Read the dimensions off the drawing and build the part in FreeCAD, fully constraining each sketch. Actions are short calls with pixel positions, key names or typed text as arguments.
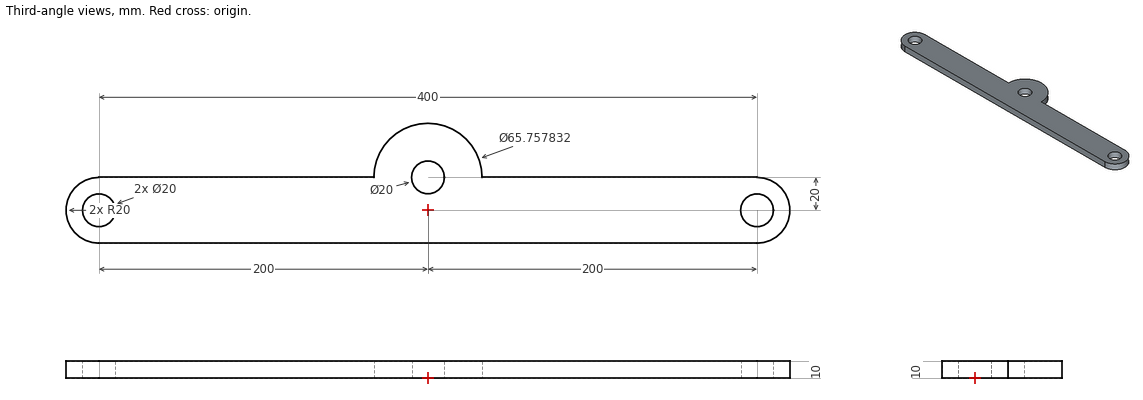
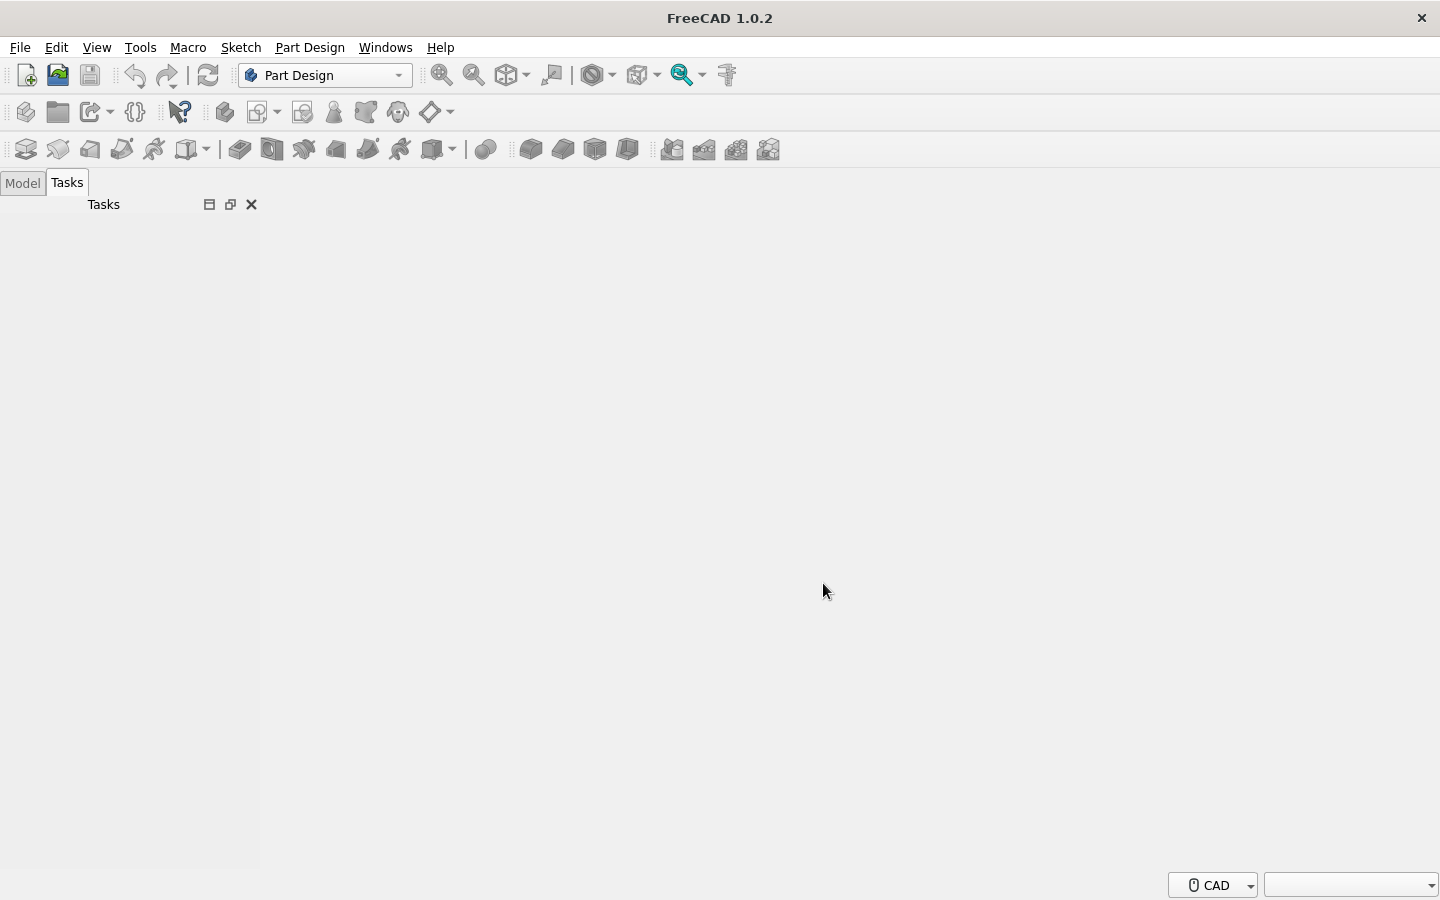
click(26, 76)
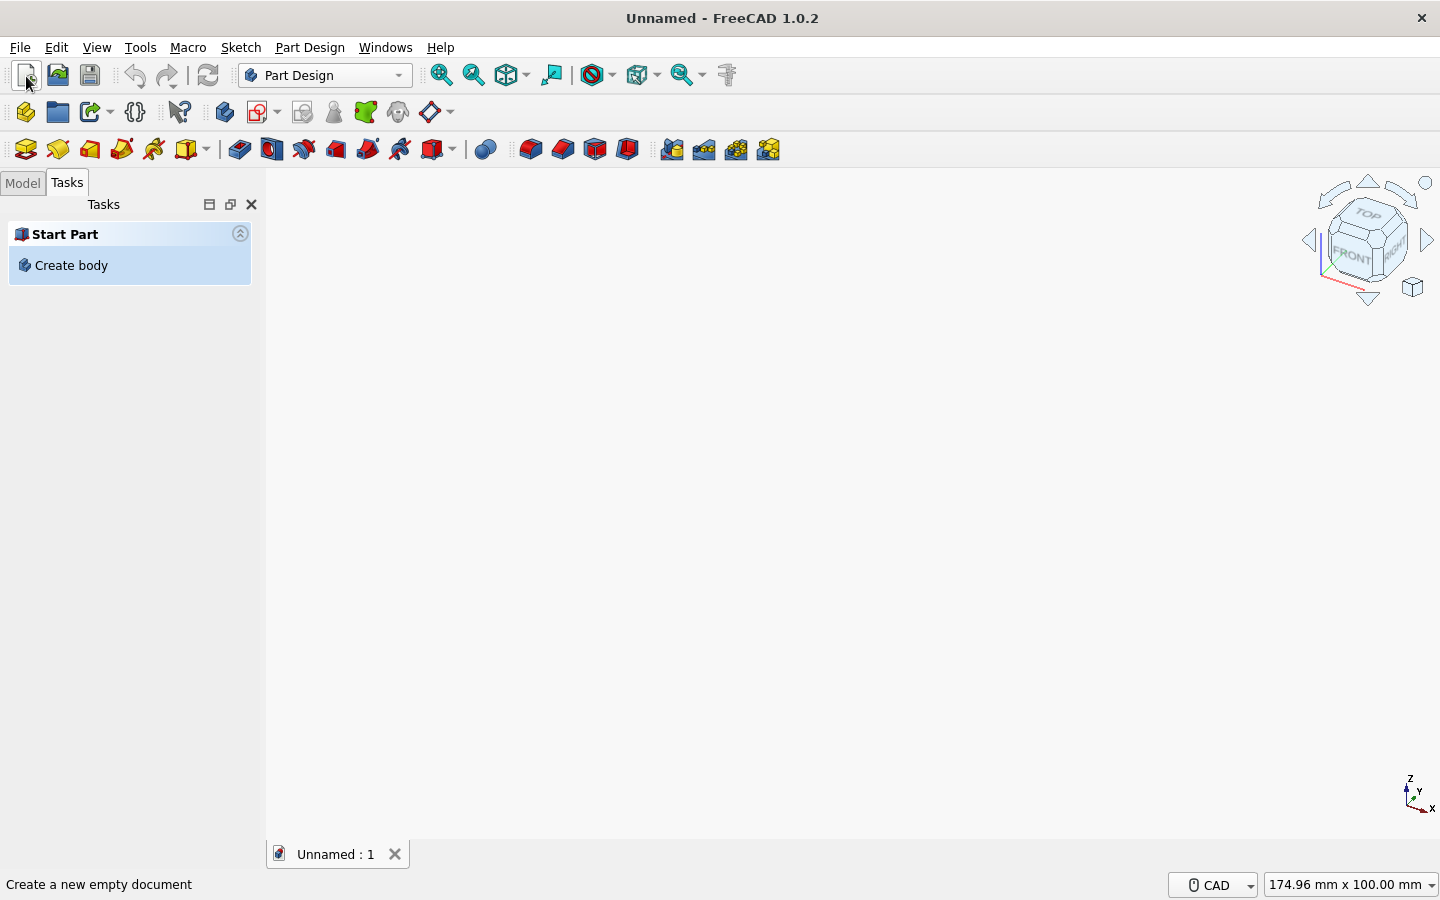
click(258, 112)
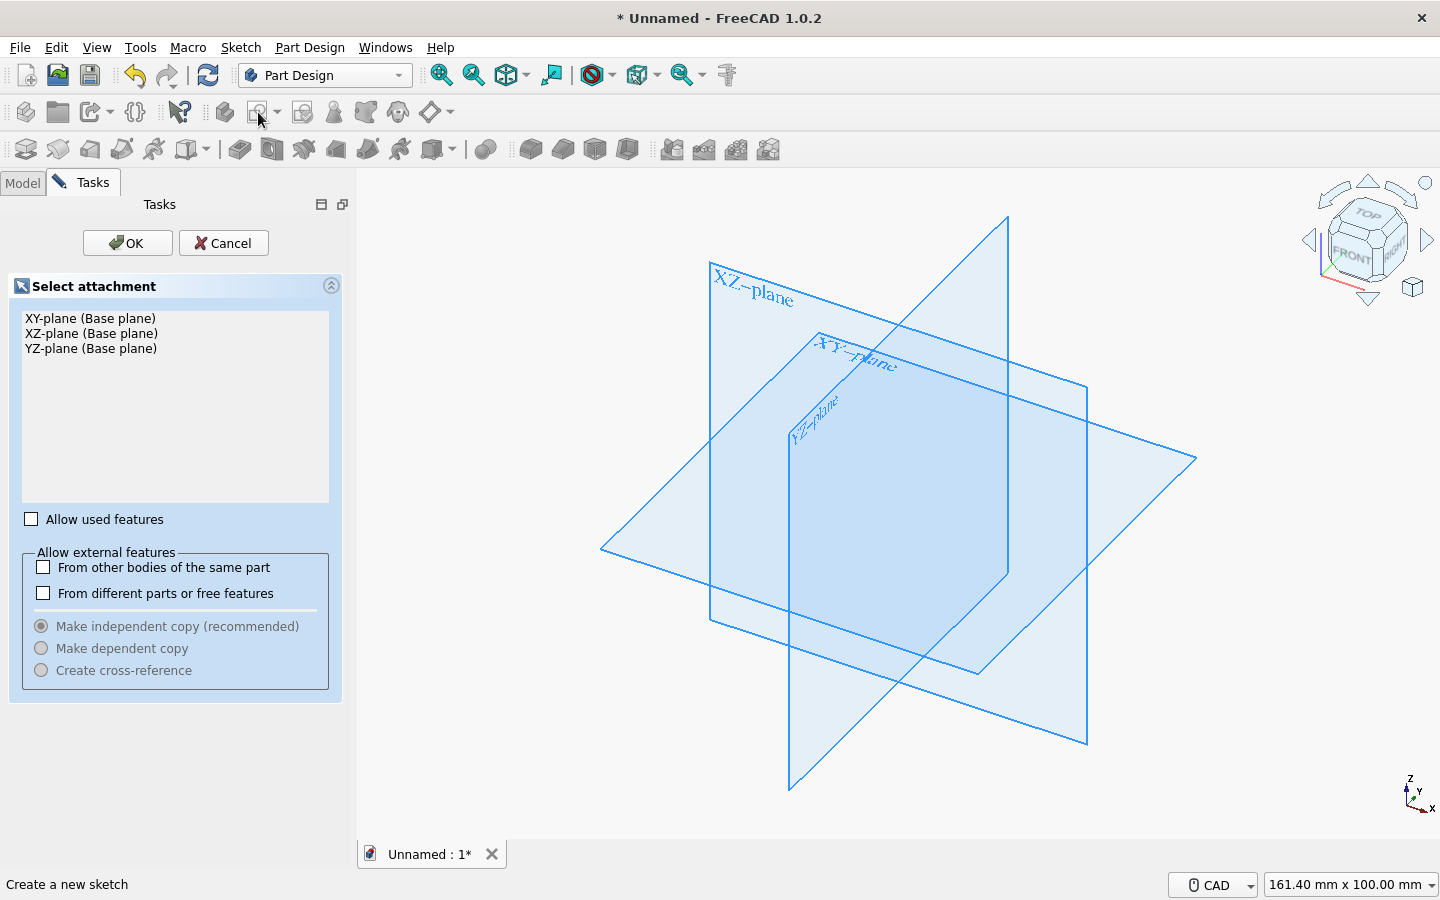
click(82, 318)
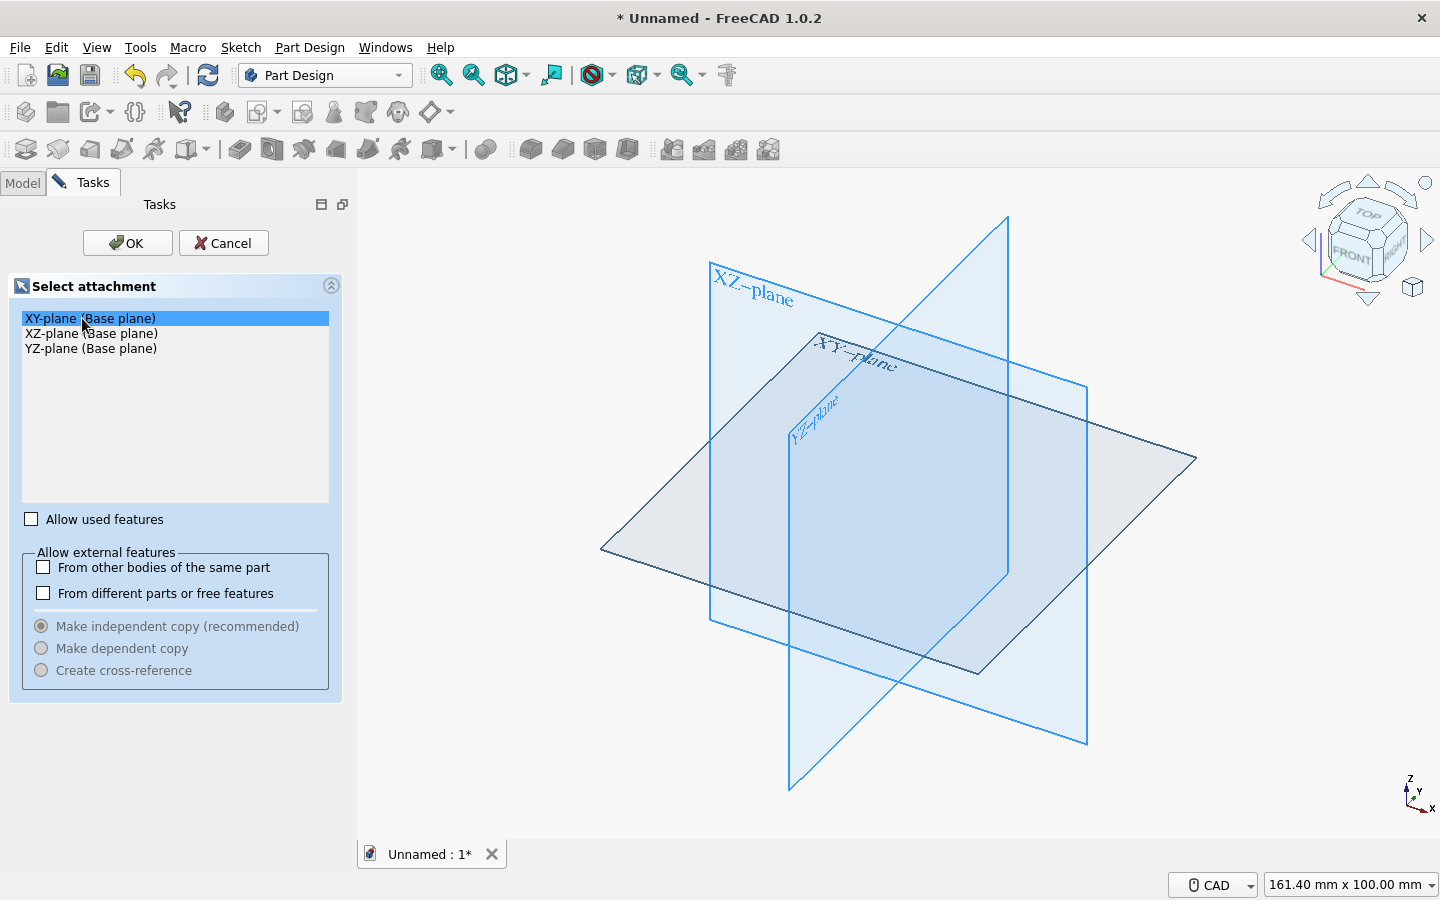
click(128, 243)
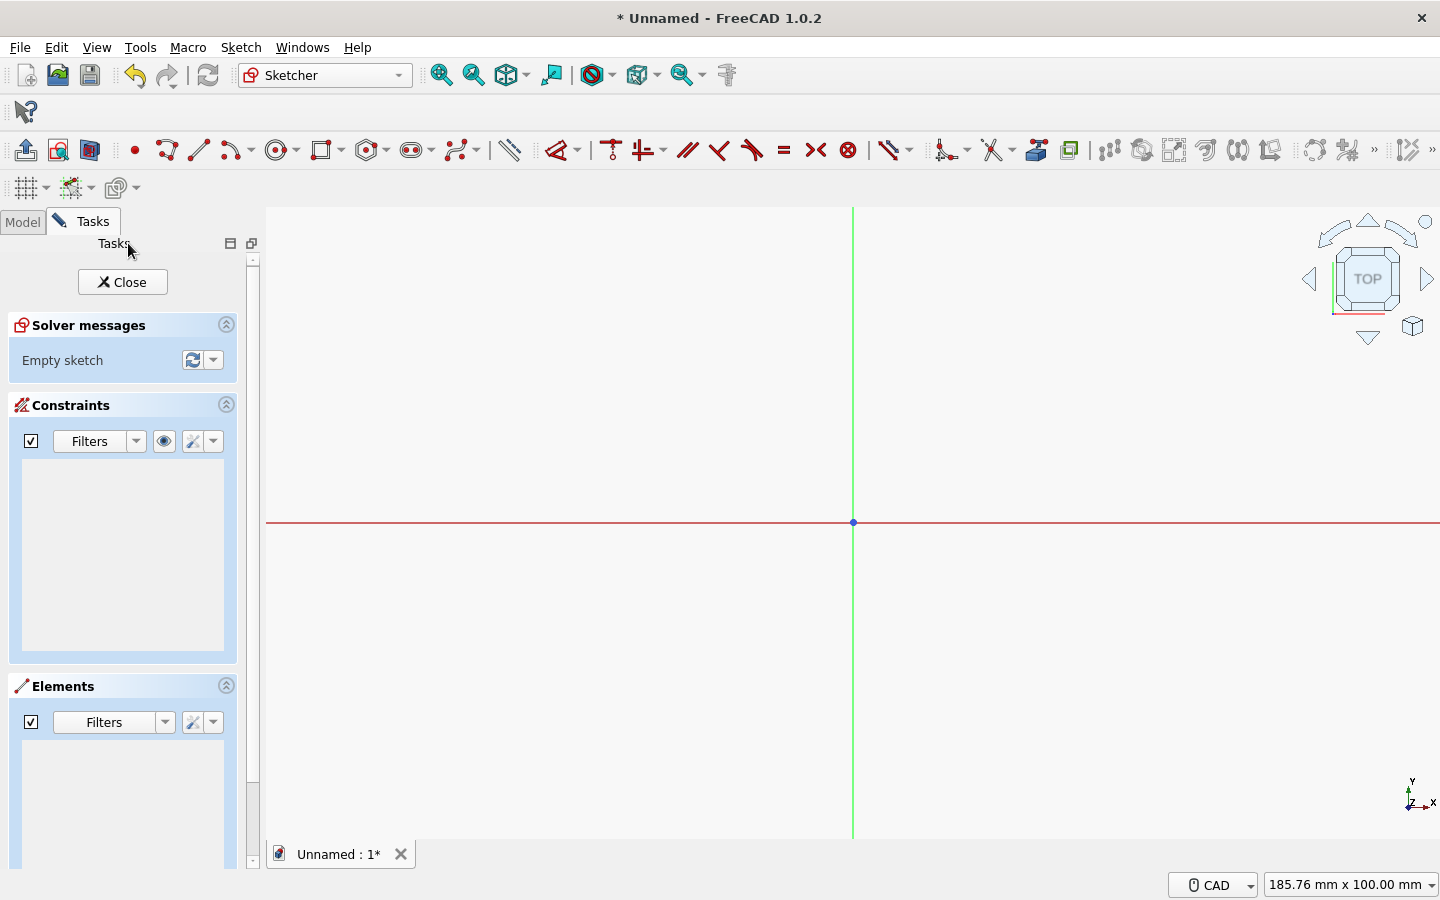
scroll(762, 523, down, 7)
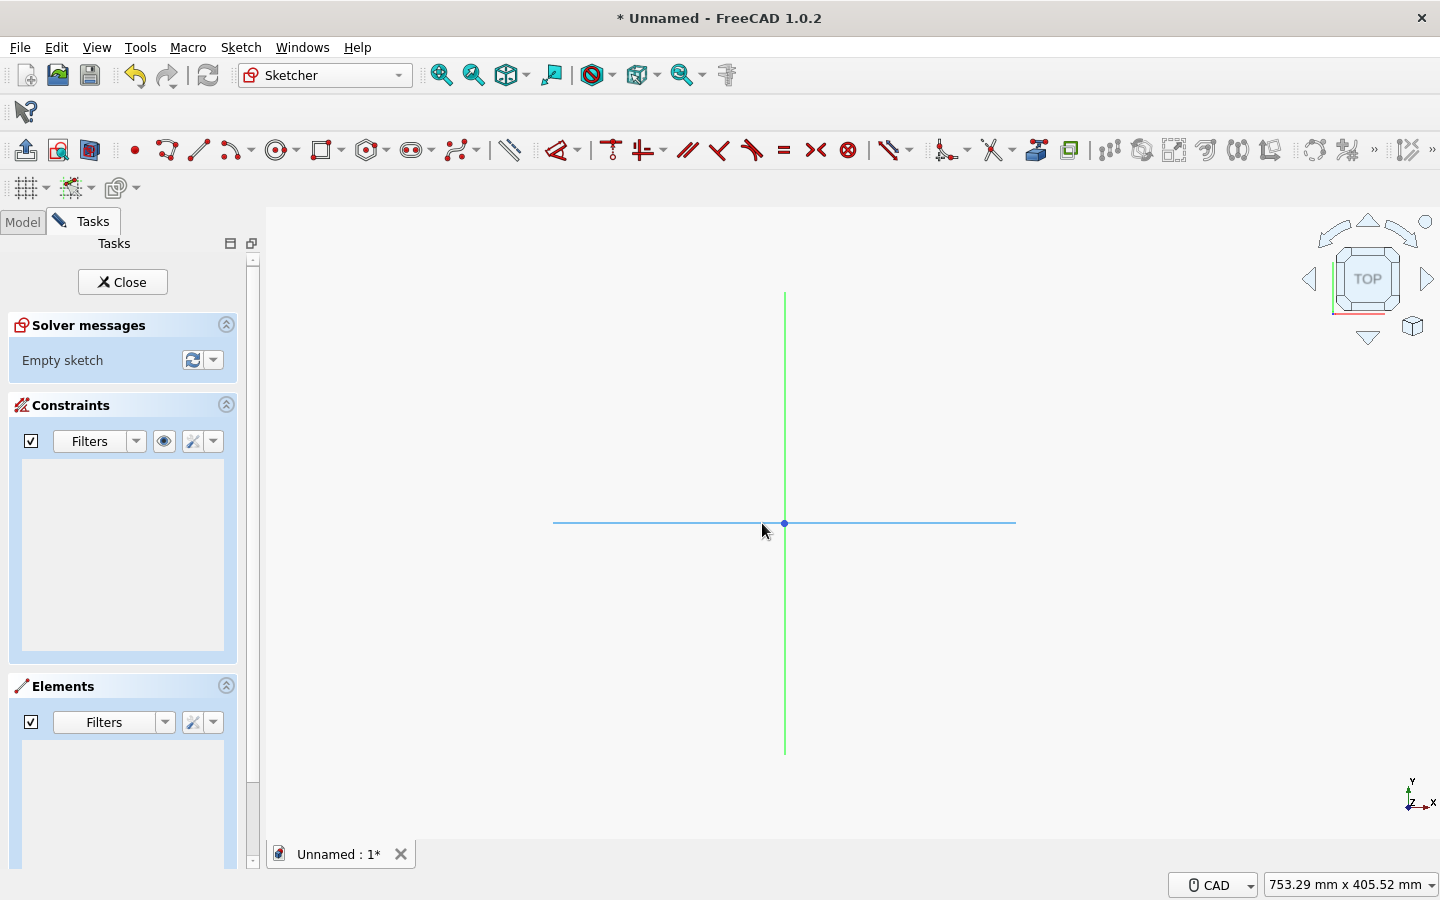
click(412, 150)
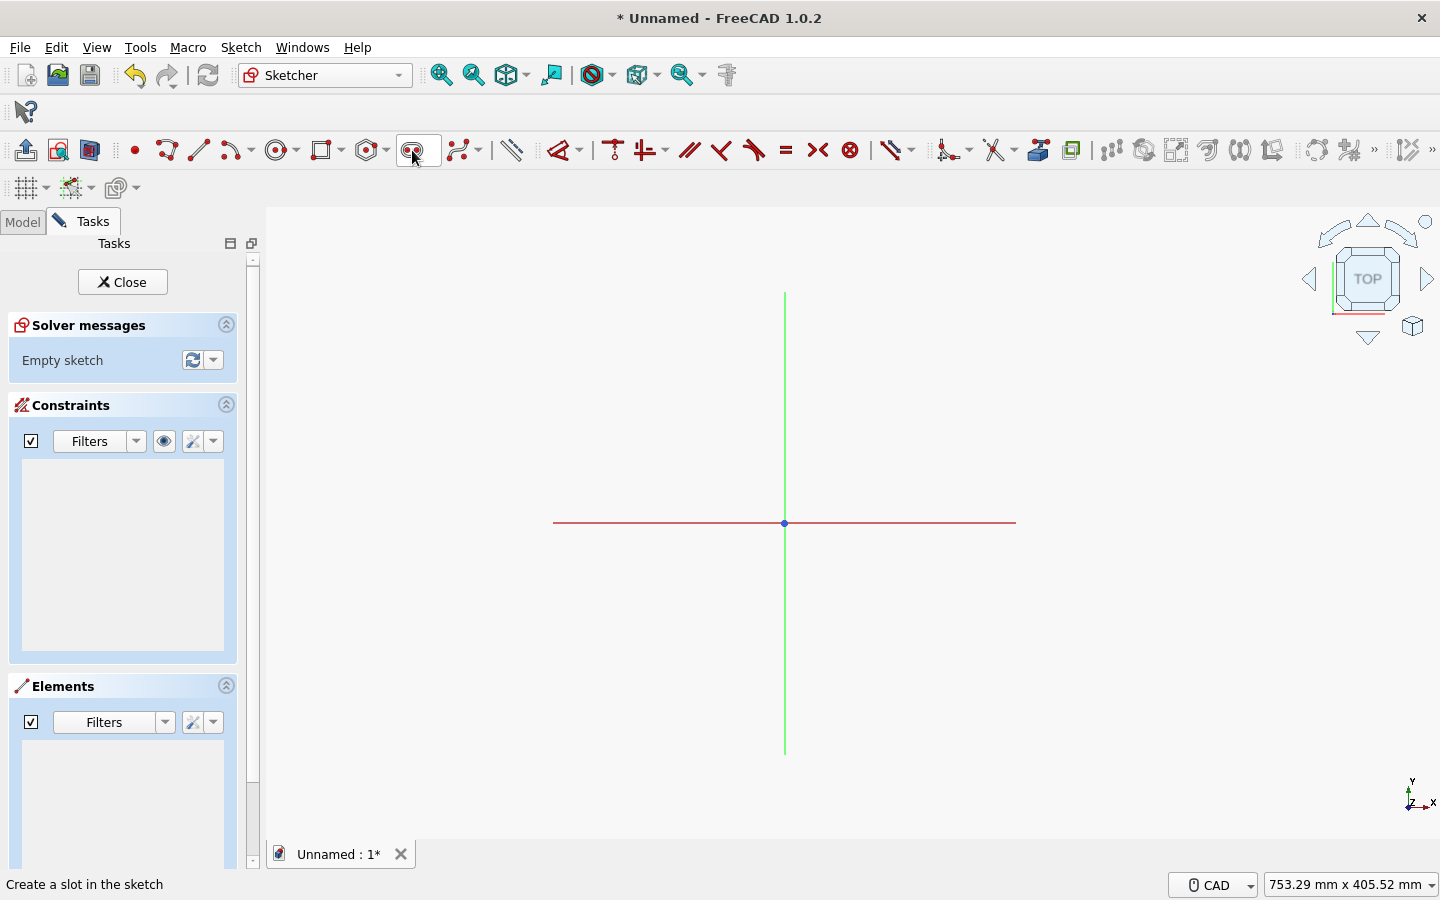
click(473, 523)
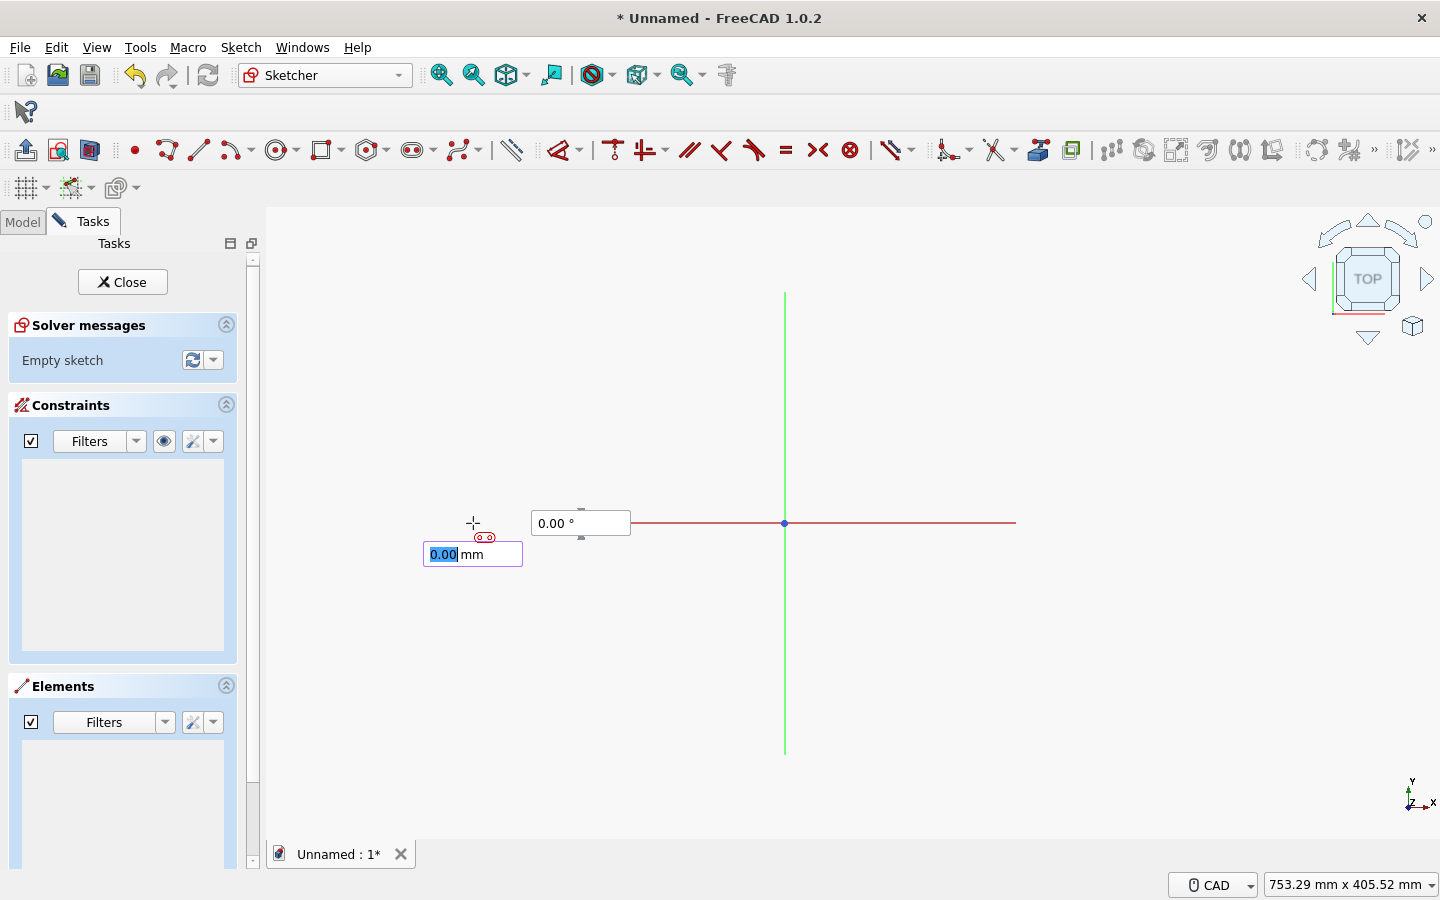
click(1096, 514)